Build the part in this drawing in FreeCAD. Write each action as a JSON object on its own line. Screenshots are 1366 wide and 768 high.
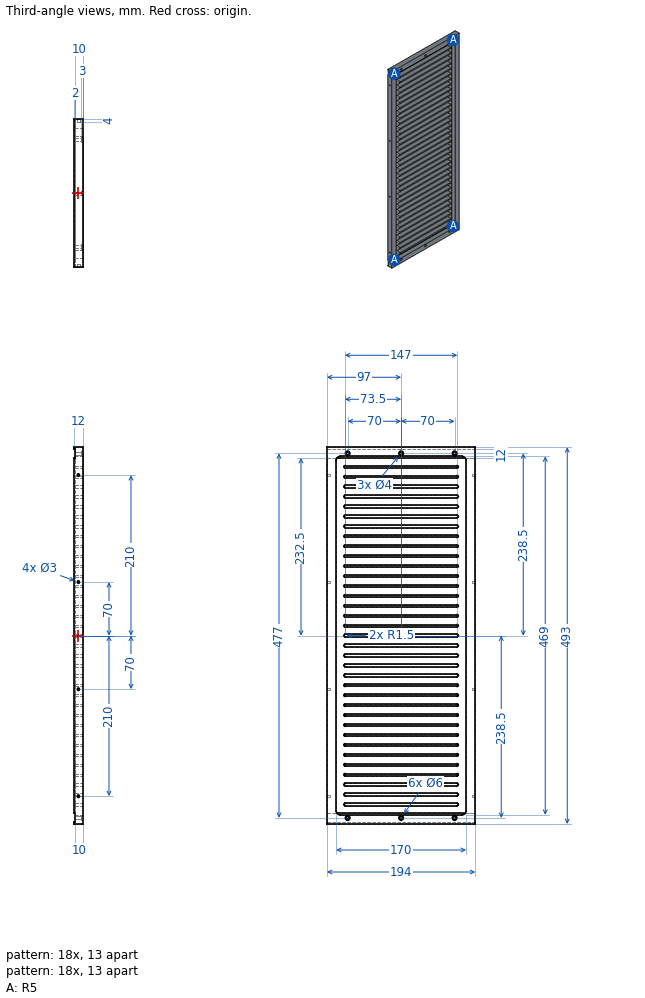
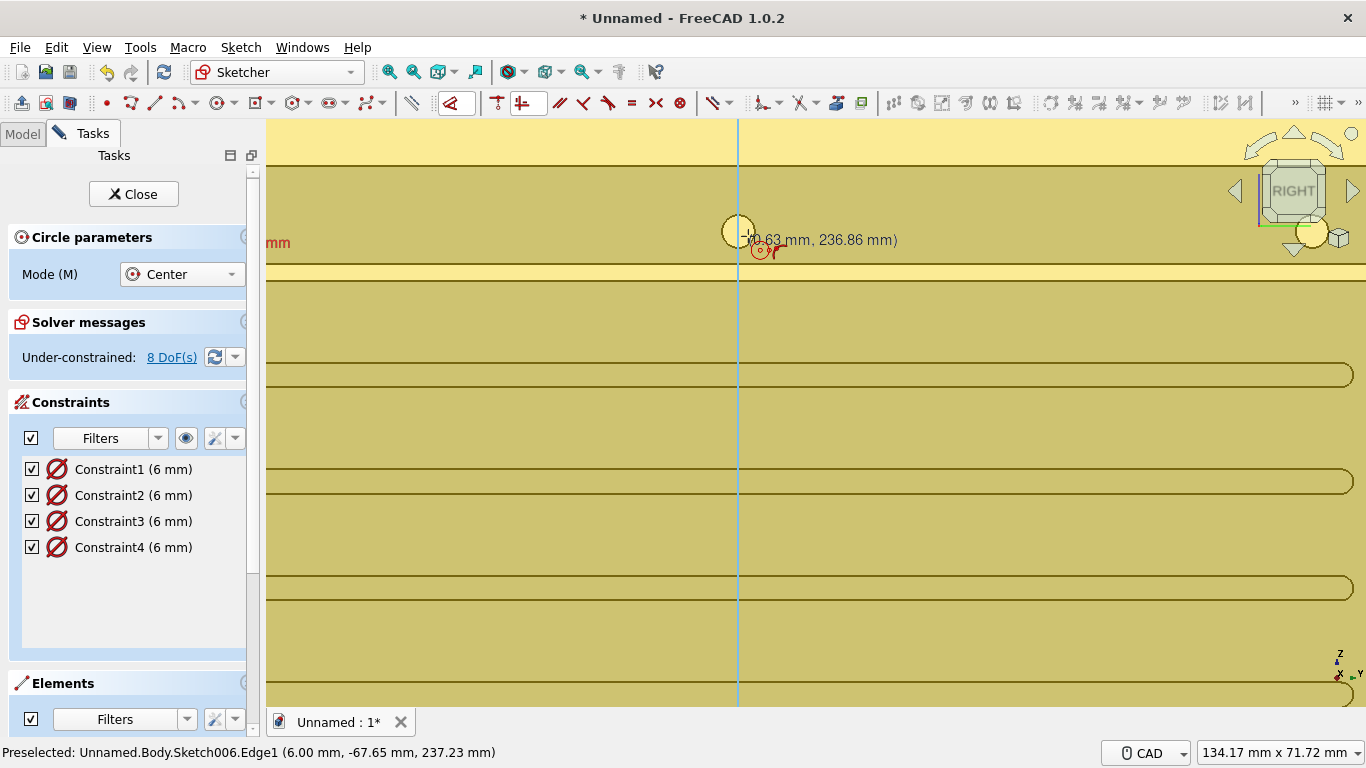
{"action": "scroll", "coordinate": [748, 236], "scroll_direction": "down", "scroll_amount": 12}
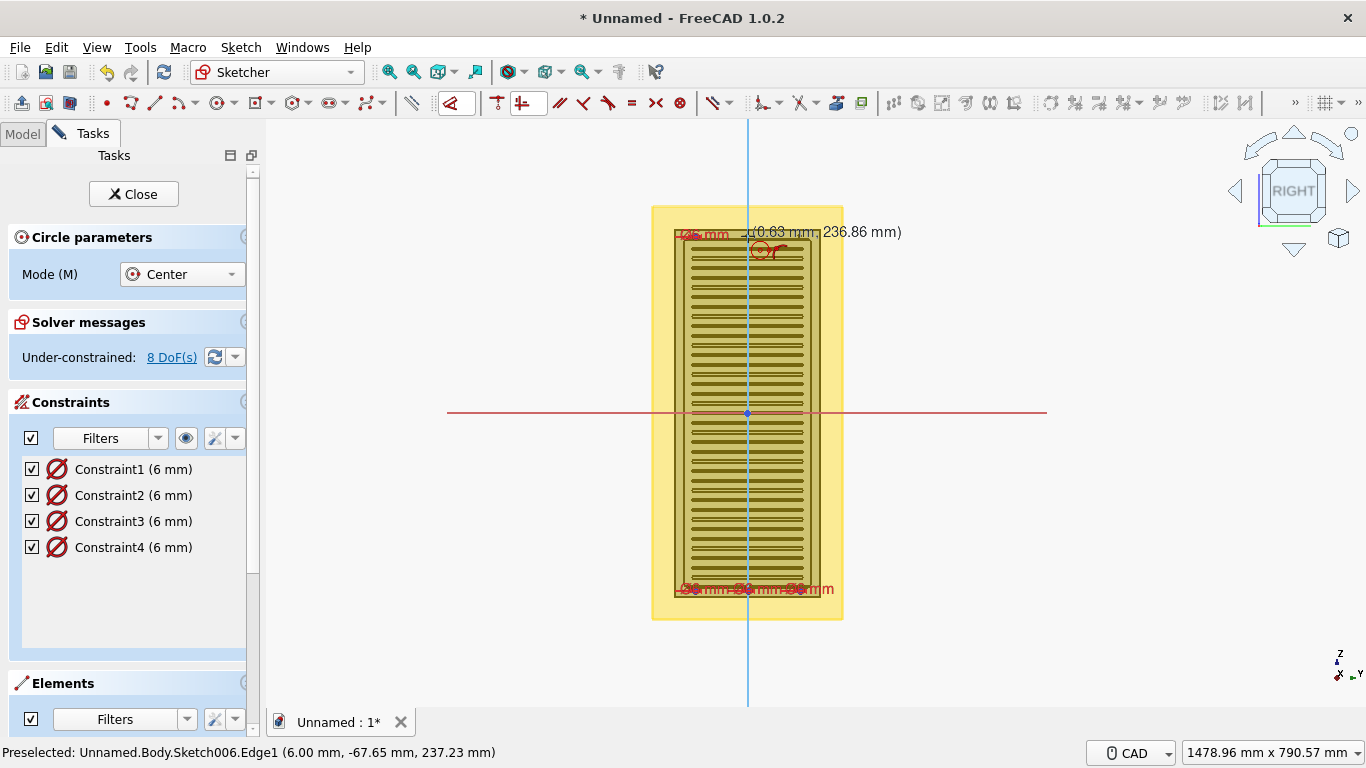
{"action": "left_click", "coordinate": [748, 236]}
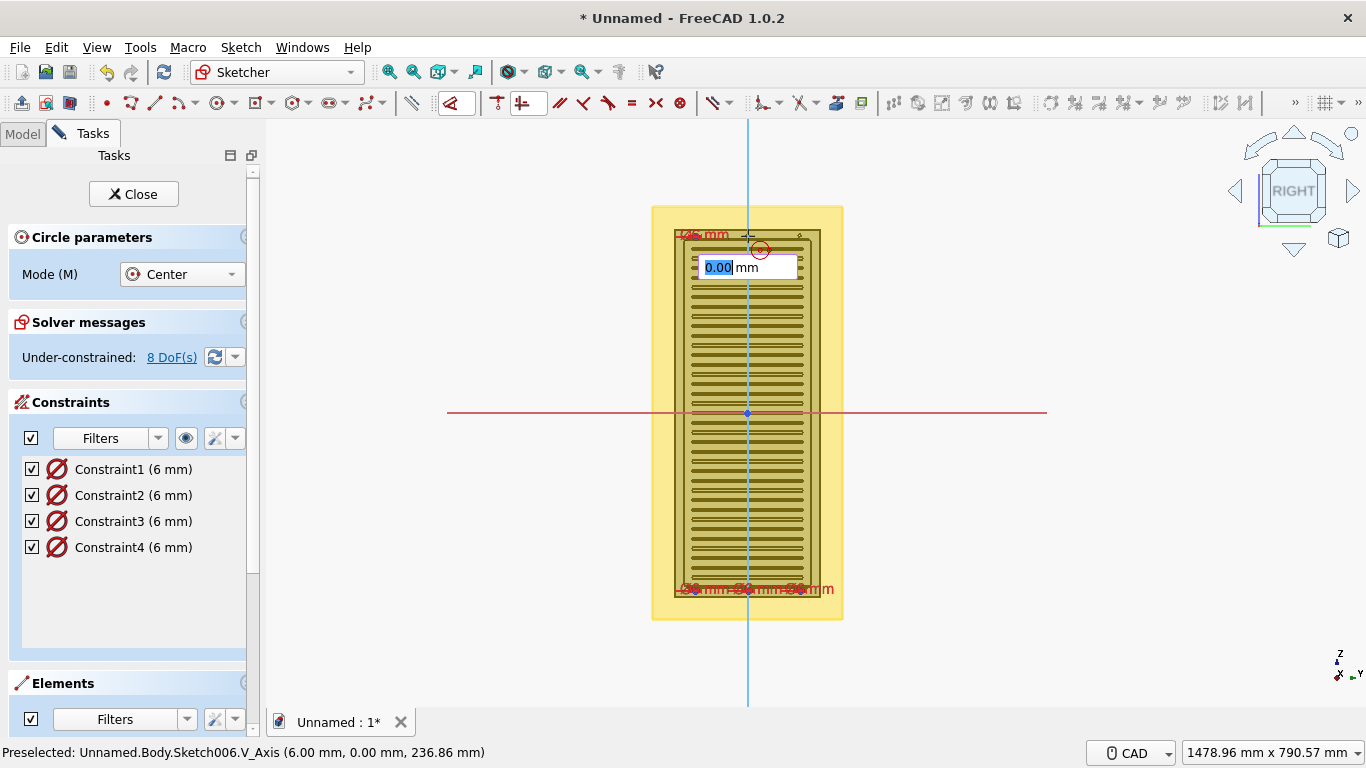
{"action": "scroll", "coordinate": [750, 235], "scroll_direction": "up", "scroll_amount": 11}
{"action": "mouse_move", "coordinate": [743, 234]}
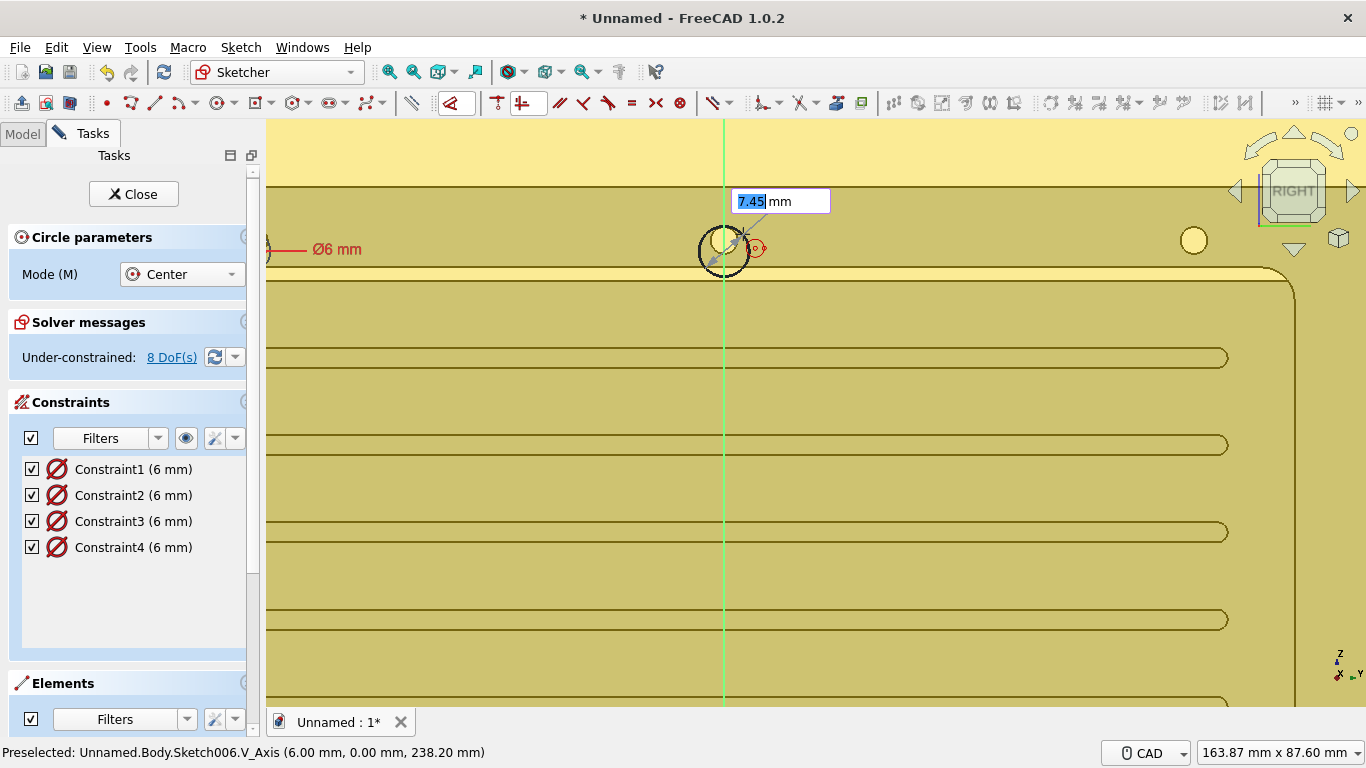
{"action": "type", "text": "6"}
{"action": "key", "text": "Return"}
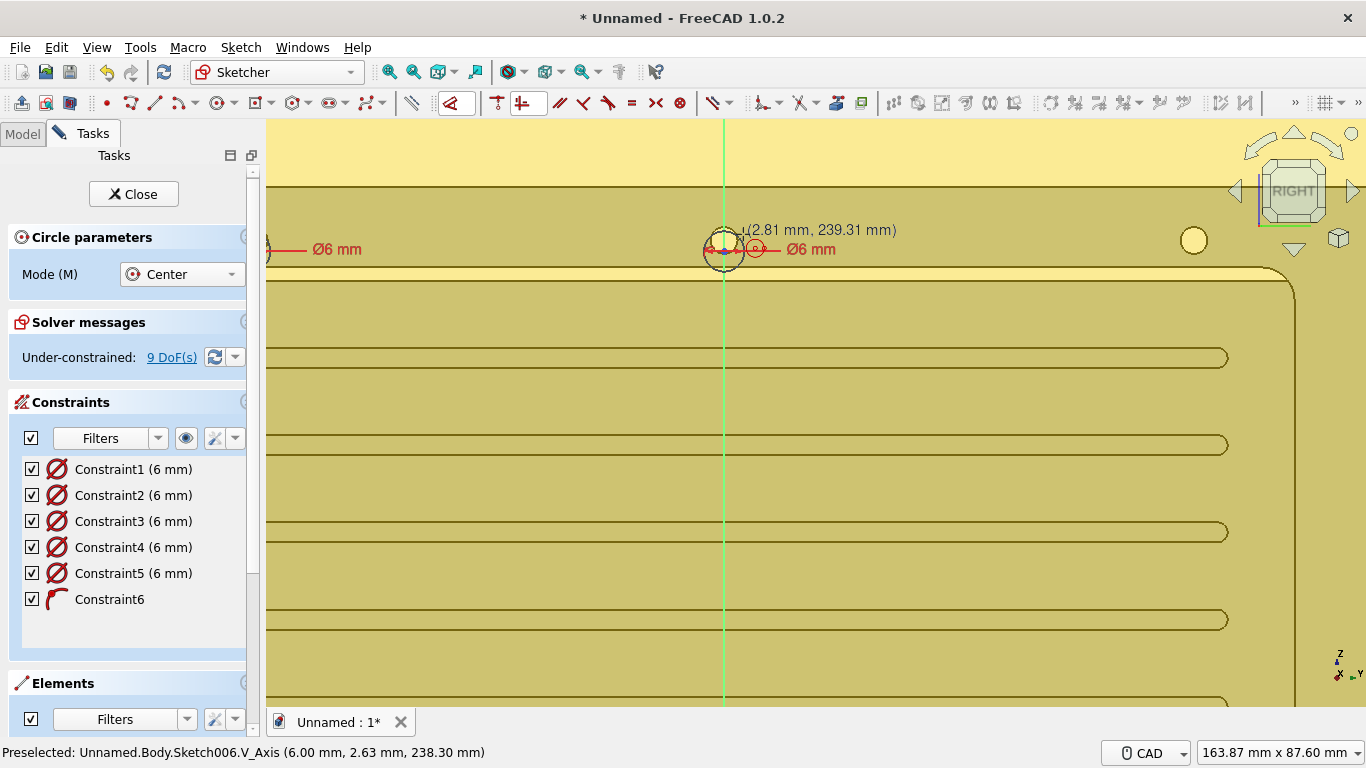
{"action": "scroll", "coordinate": [750, 235], "scroll_direction": "down", "scroll_amount": 11}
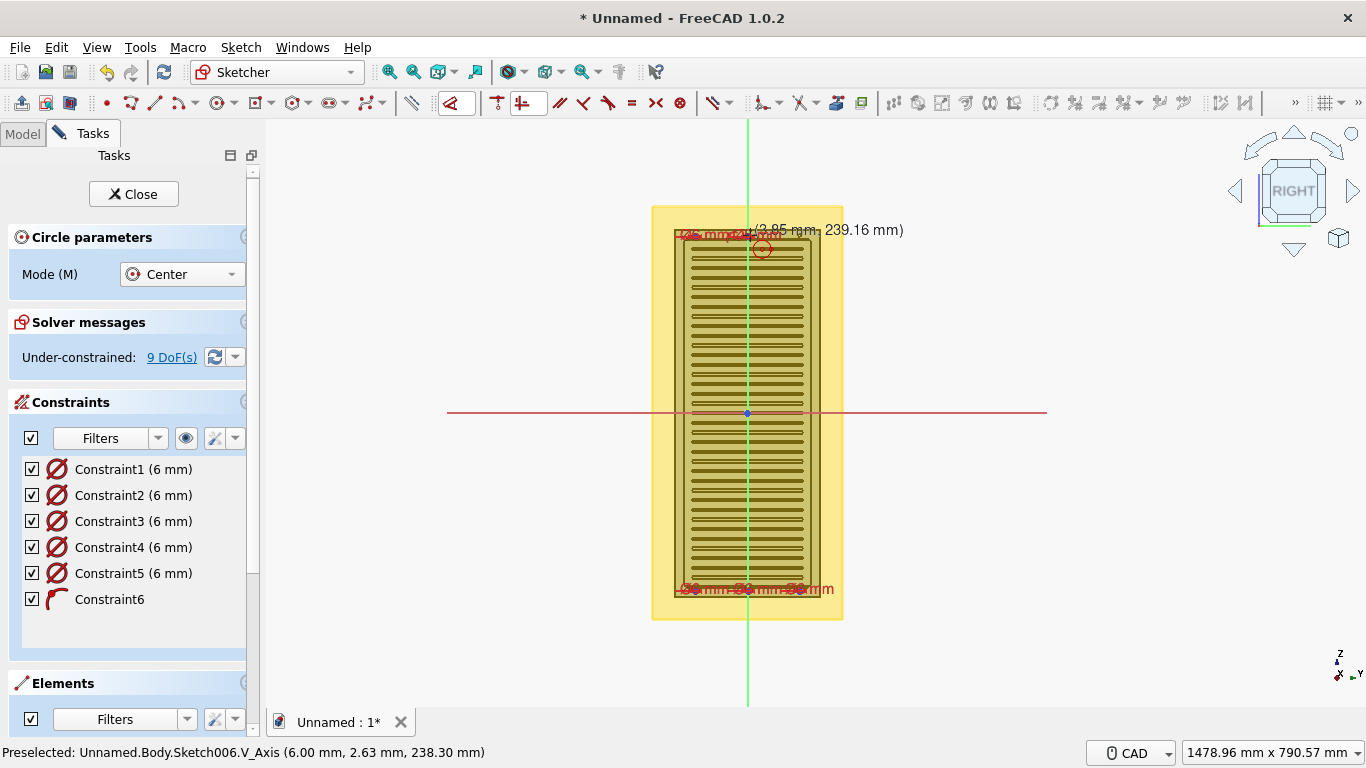
{"action": "left_click", "coordinate": [800, 236]}
{"action": "mouse_move", "coordinate": [801, 234]}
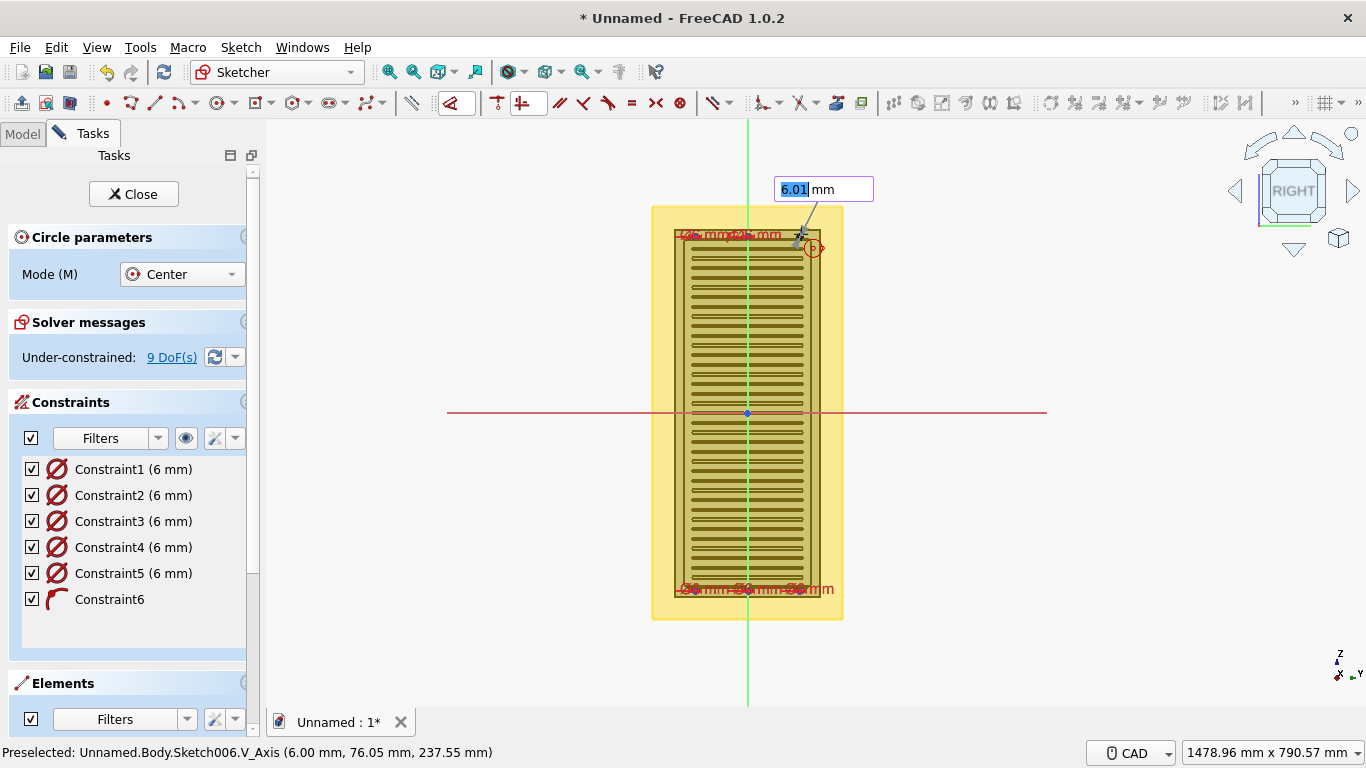
{"action": "type", "text": "6"}
{"action": "key", "text": "Return"}
{"action": "key", "text": "Escape"}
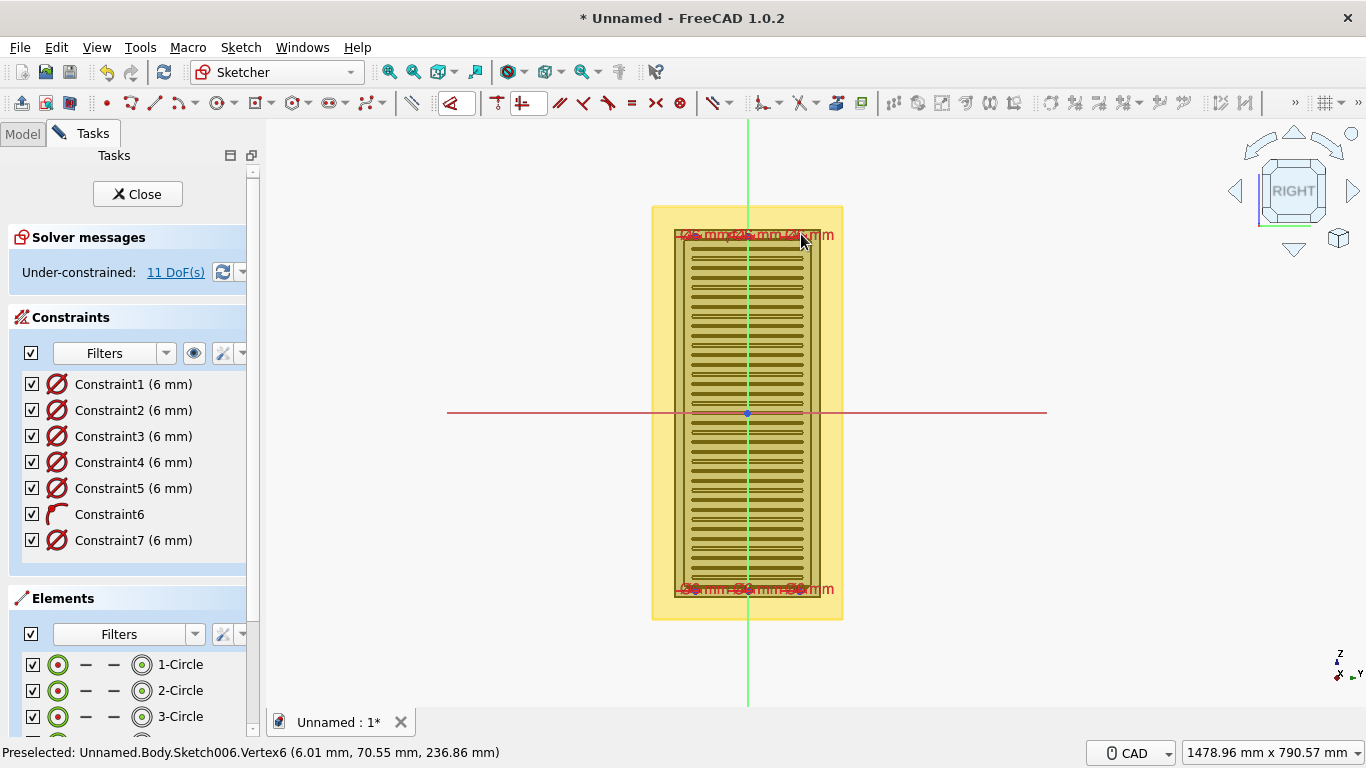
{"action": "left_click", "coordinate": [748, 591]}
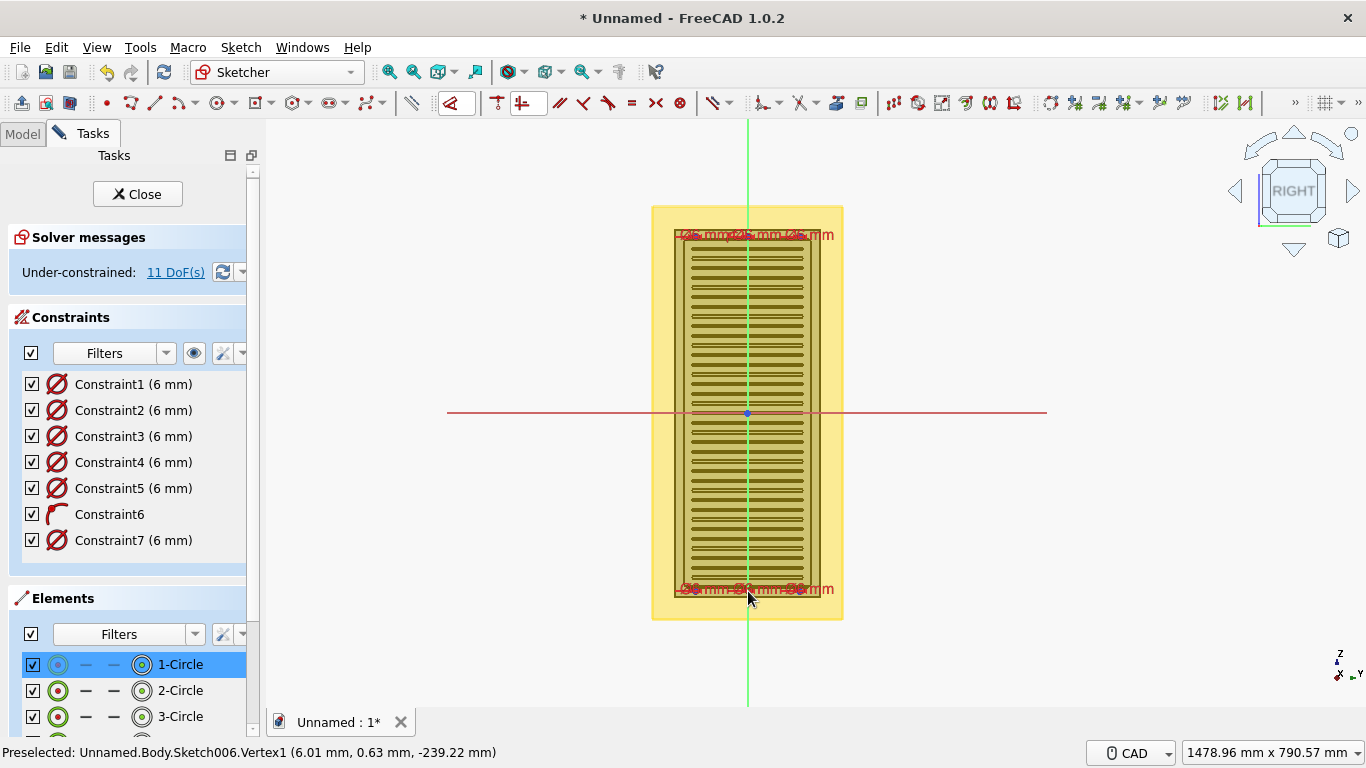
{"action": "left_click", "coordinate": [748, 641]}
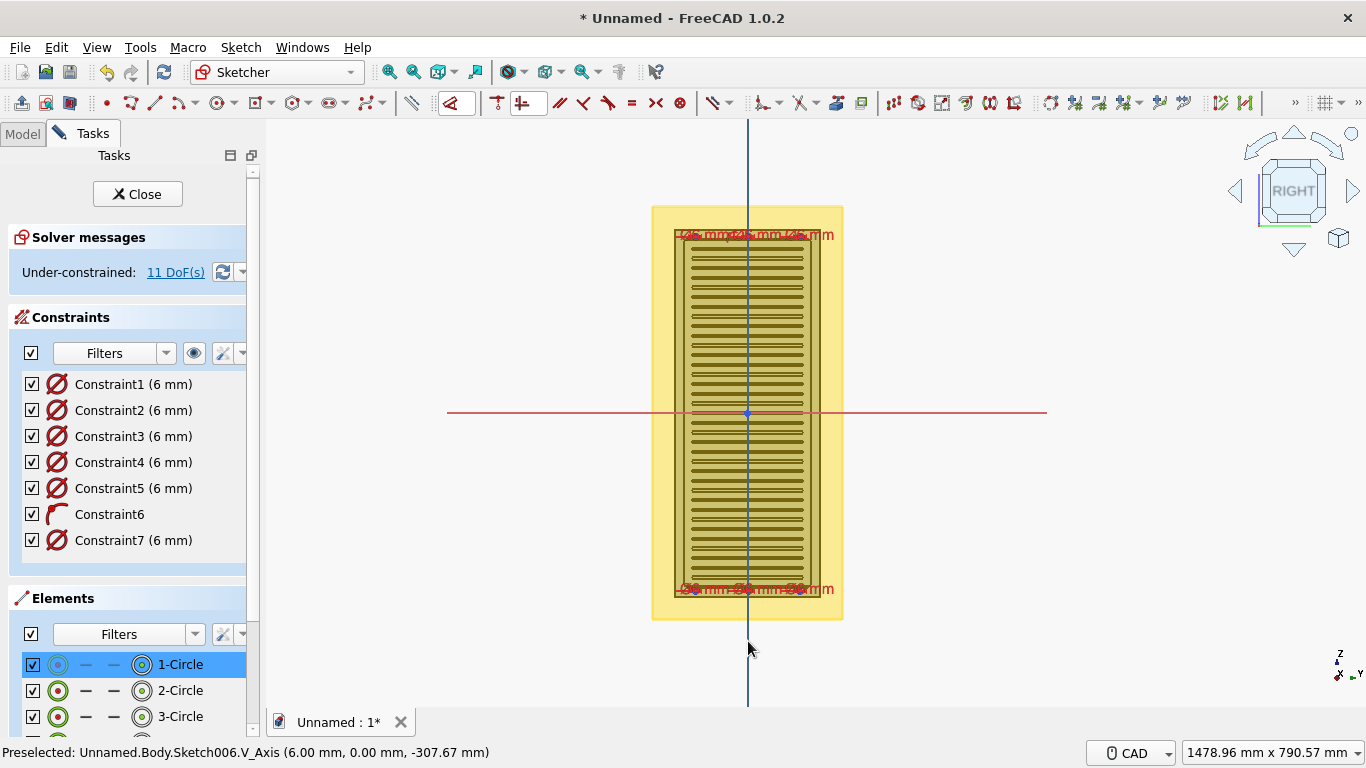
{"action": "left_click", "coordinate": [498, 104]}